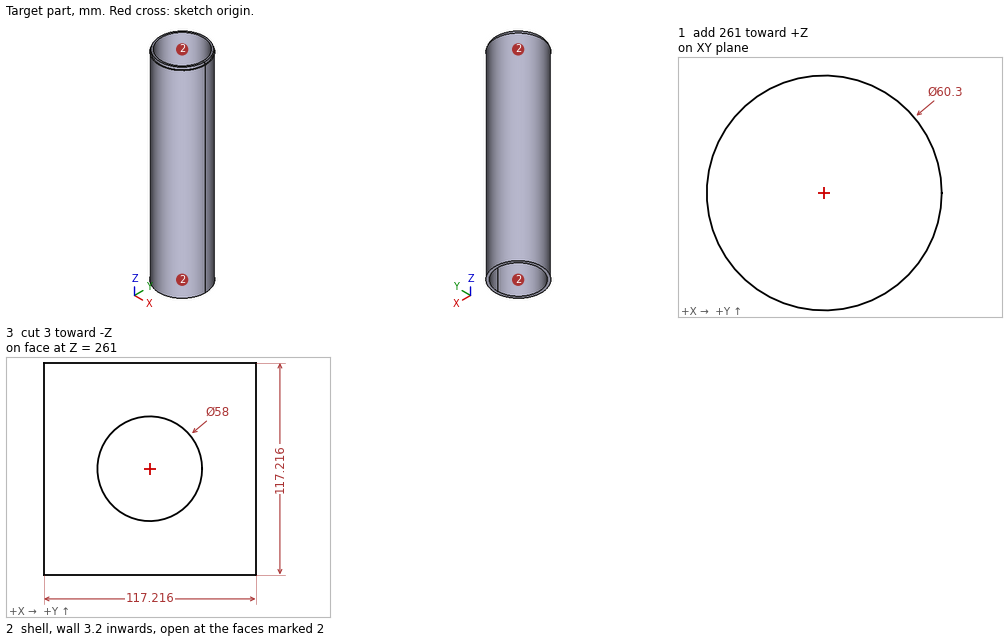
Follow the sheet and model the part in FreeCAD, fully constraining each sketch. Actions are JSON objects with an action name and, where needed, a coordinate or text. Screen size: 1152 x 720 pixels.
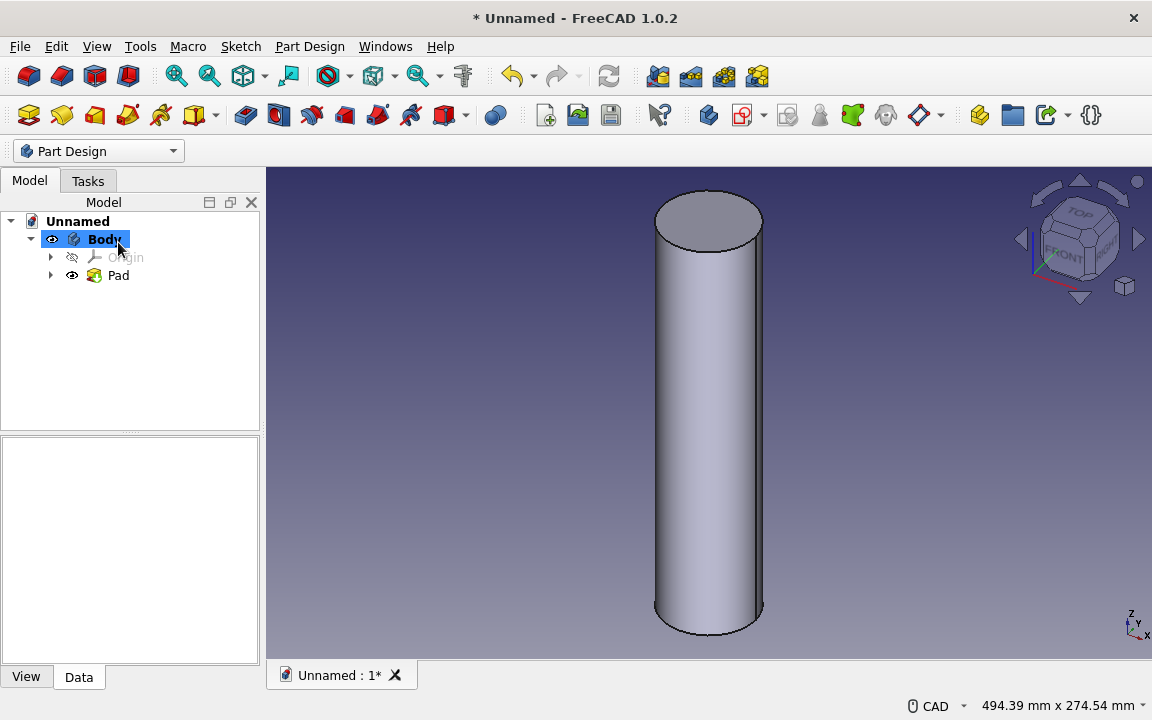
{"action": "left_click", "coordinate": [709, 220]}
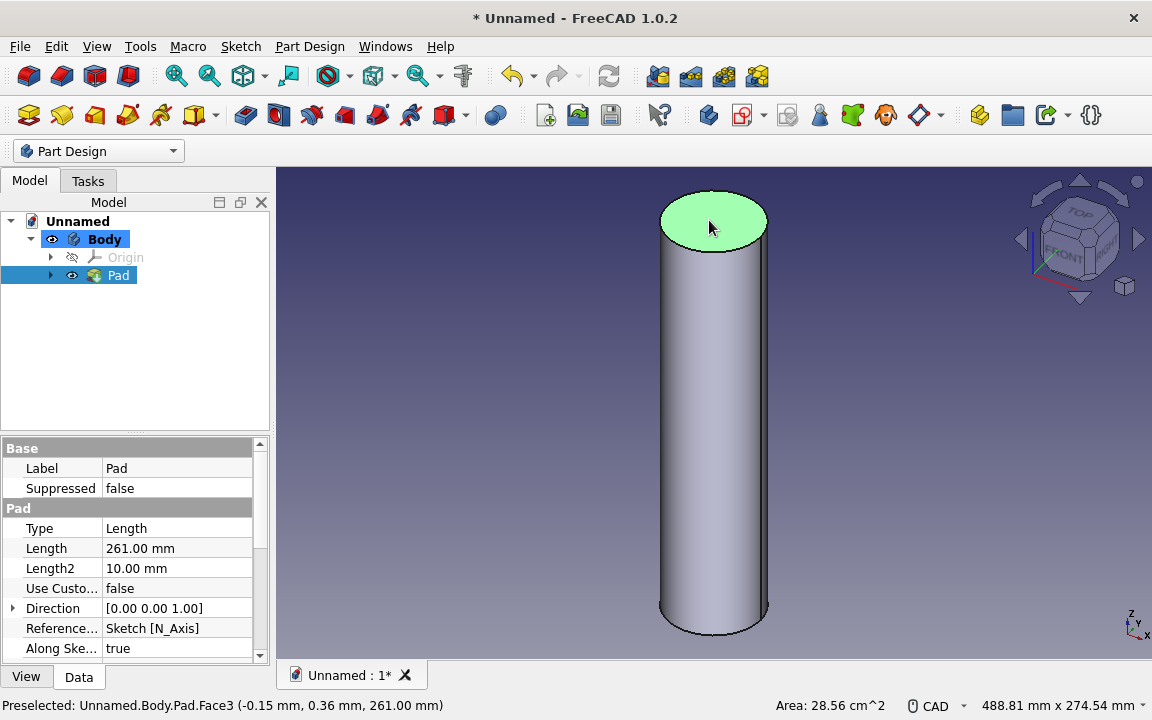
{"action": "key", "text": "0"}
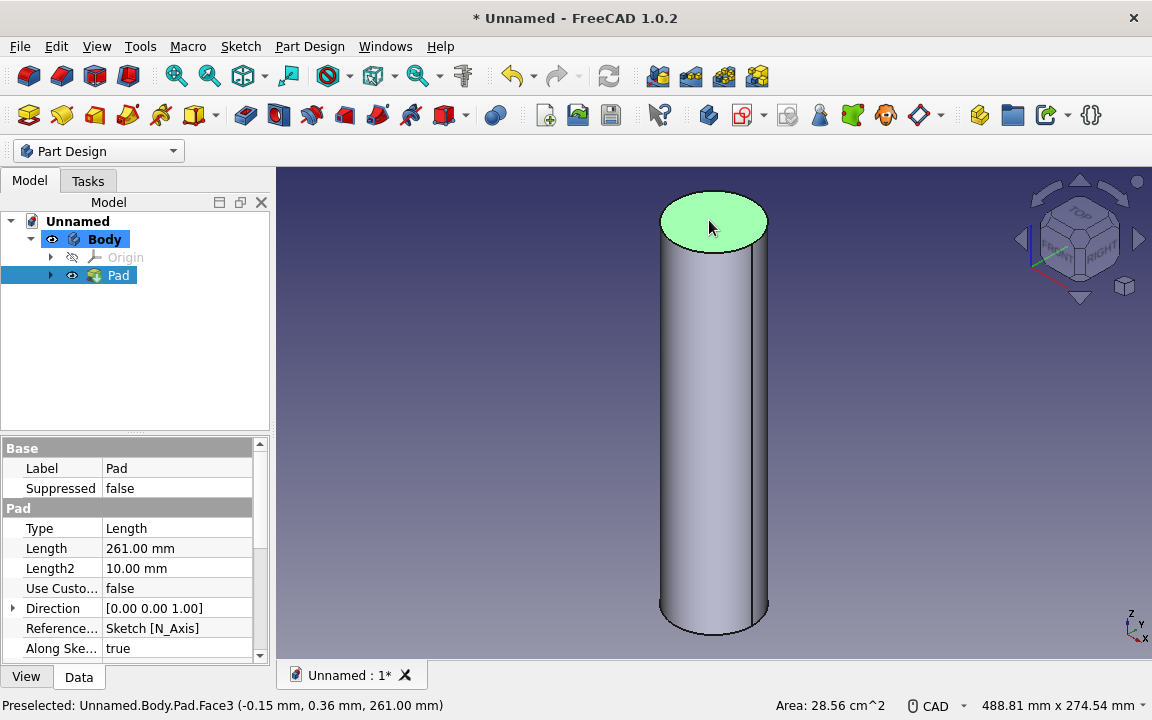
{"action": "key", "text": "2"}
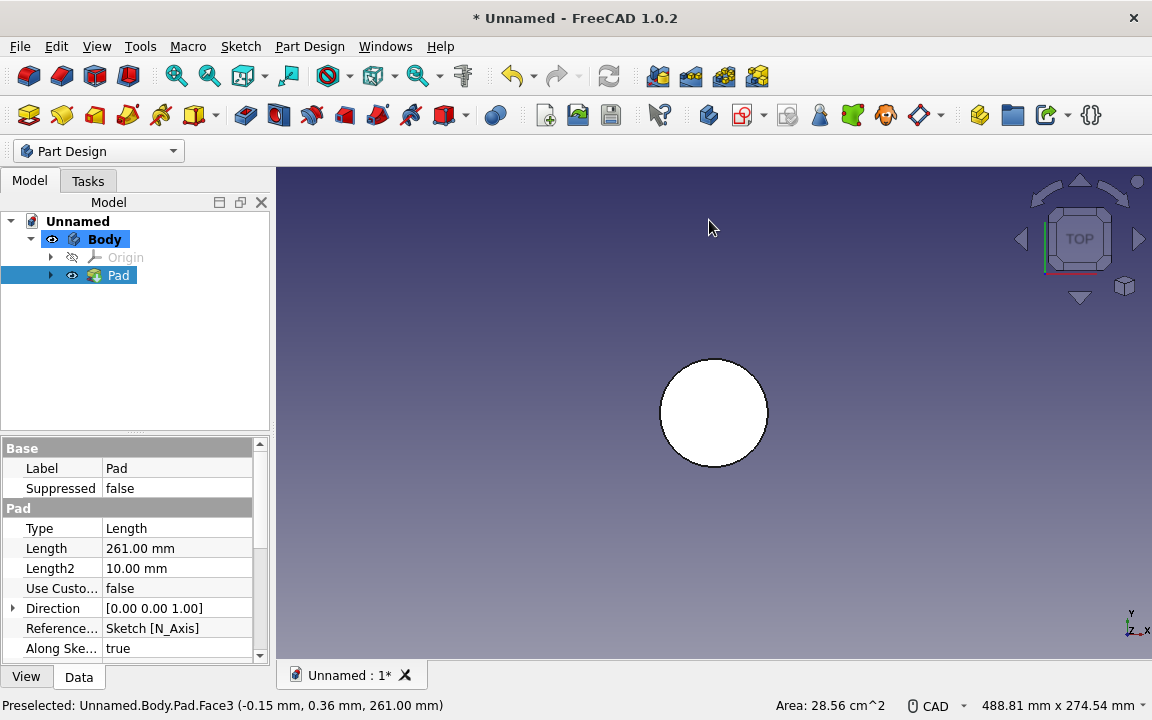
{"action": "left_click", "coordinate": [177, 76]}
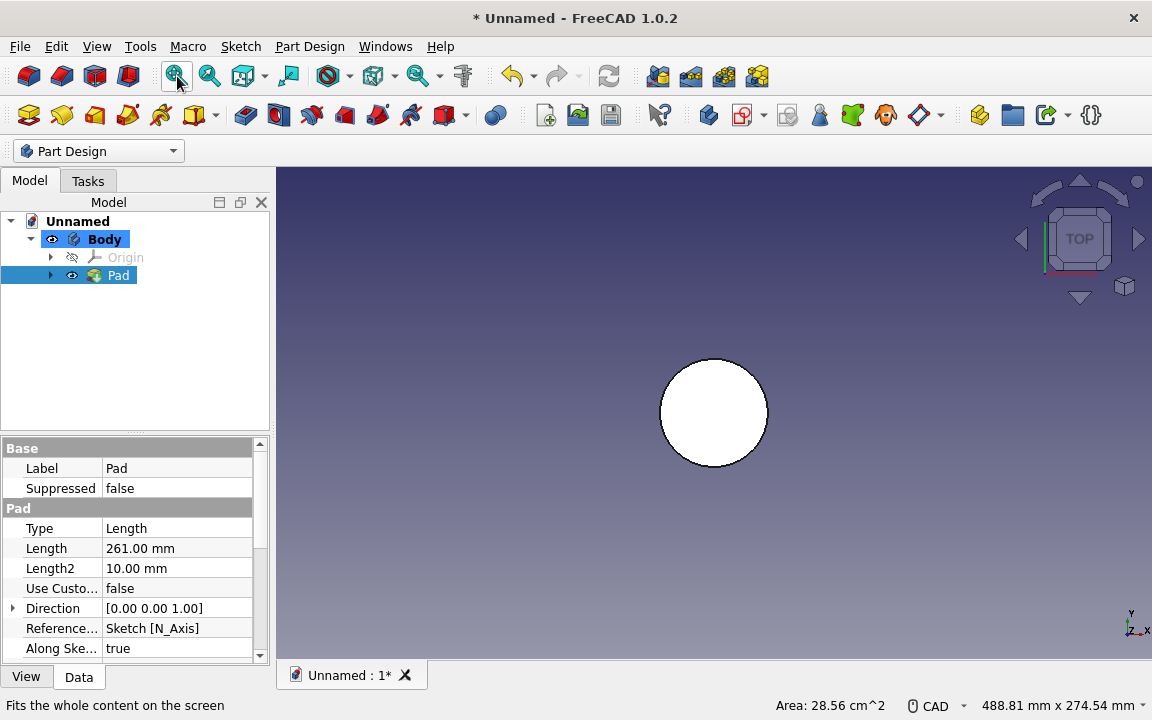
{"action": "key", "text": "1"}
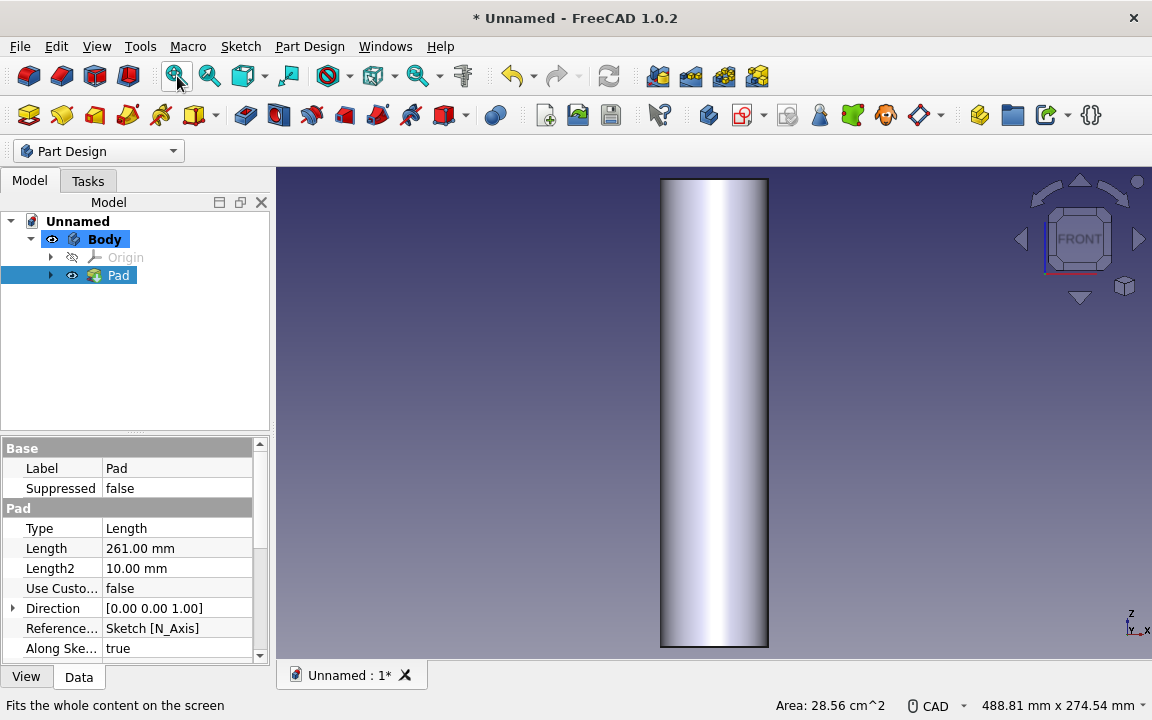
{"action": "key", "text": "3"}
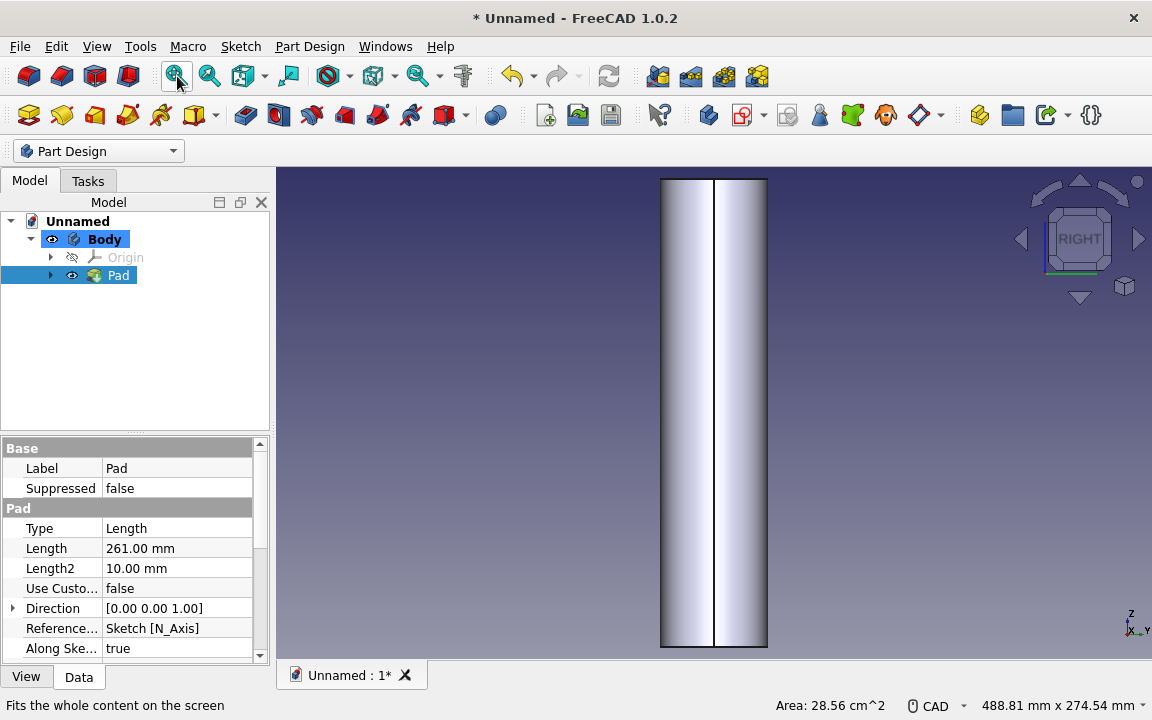
{"action": "key", "text": "5"}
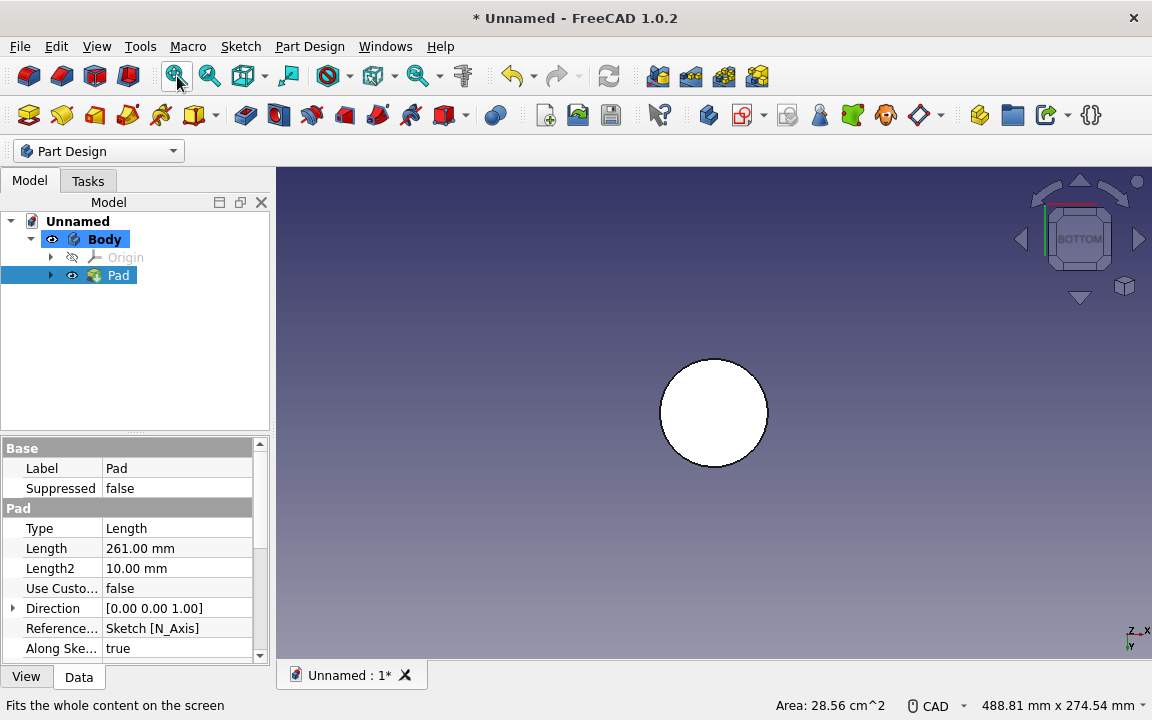
{"action": "key", "text": "v f"}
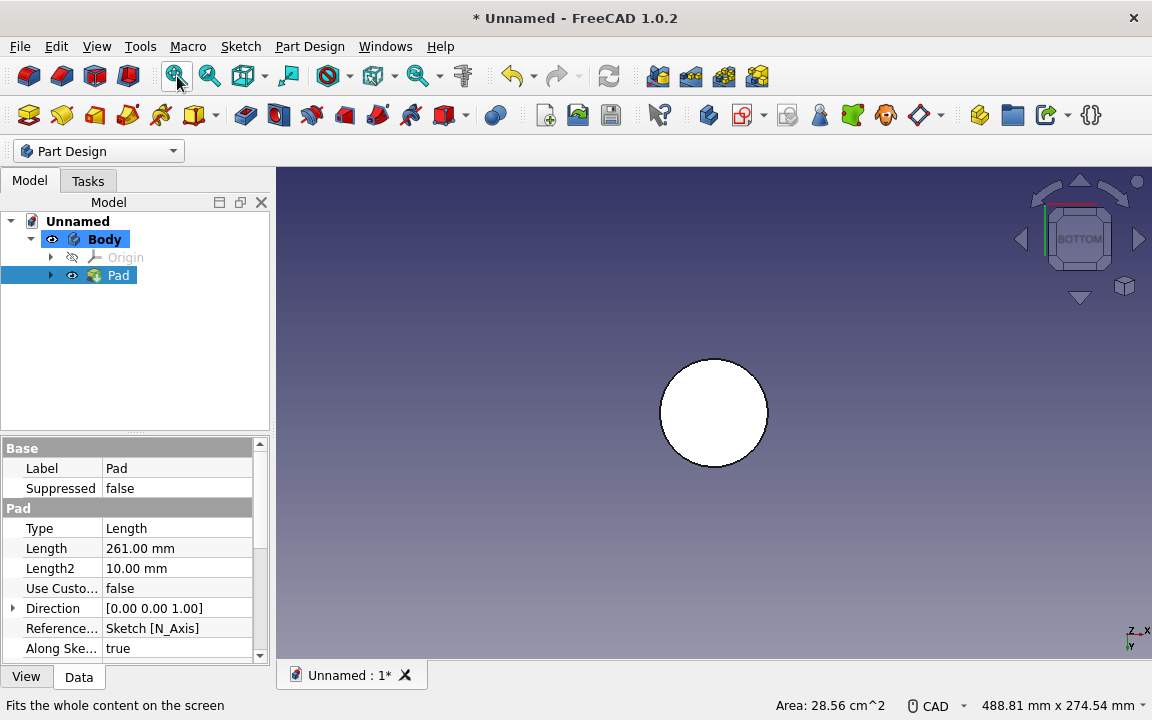
{"action": "left_click", "coordinate": [714, 412], "text": "ctrl"}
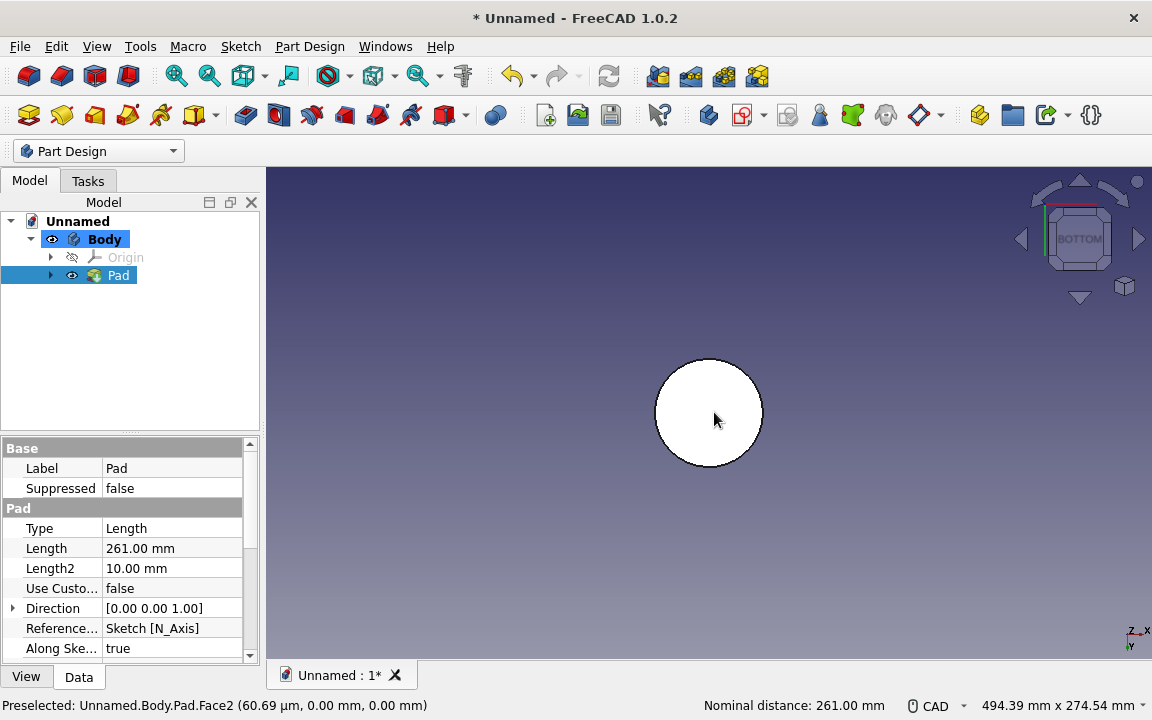
{"action": "left_click", "coordinate": [128, 76]}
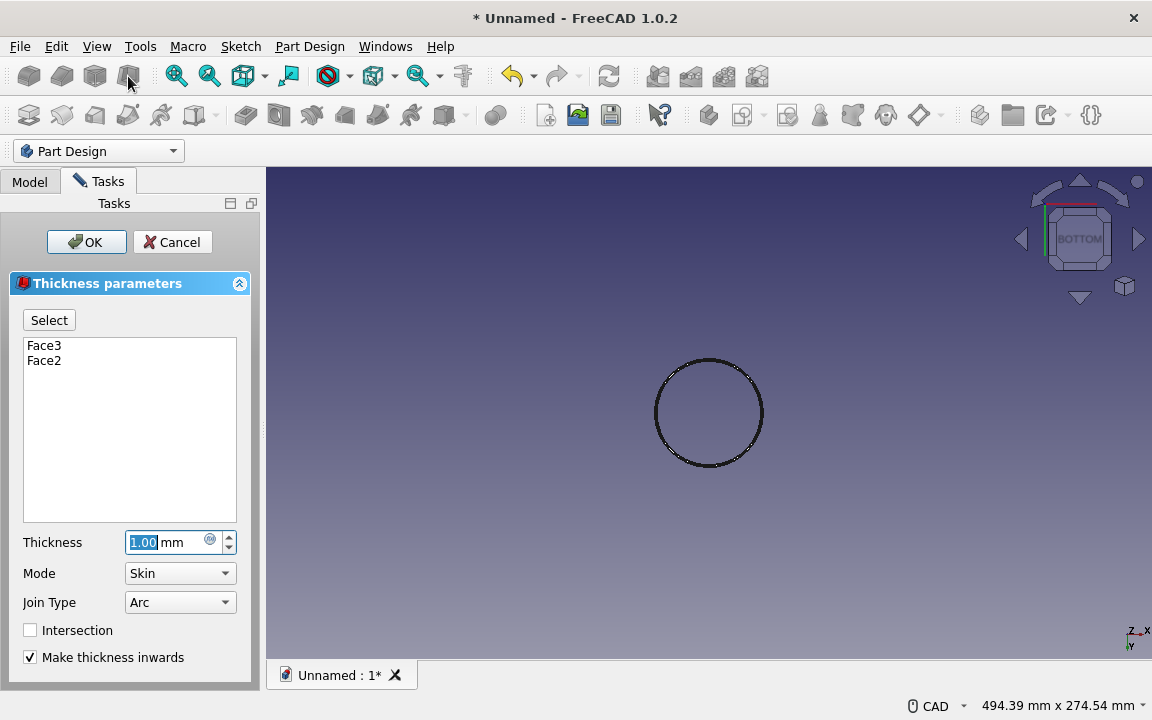
{"action": "type", "text": "3.2"}
{"action": "key", "text": "Tab"}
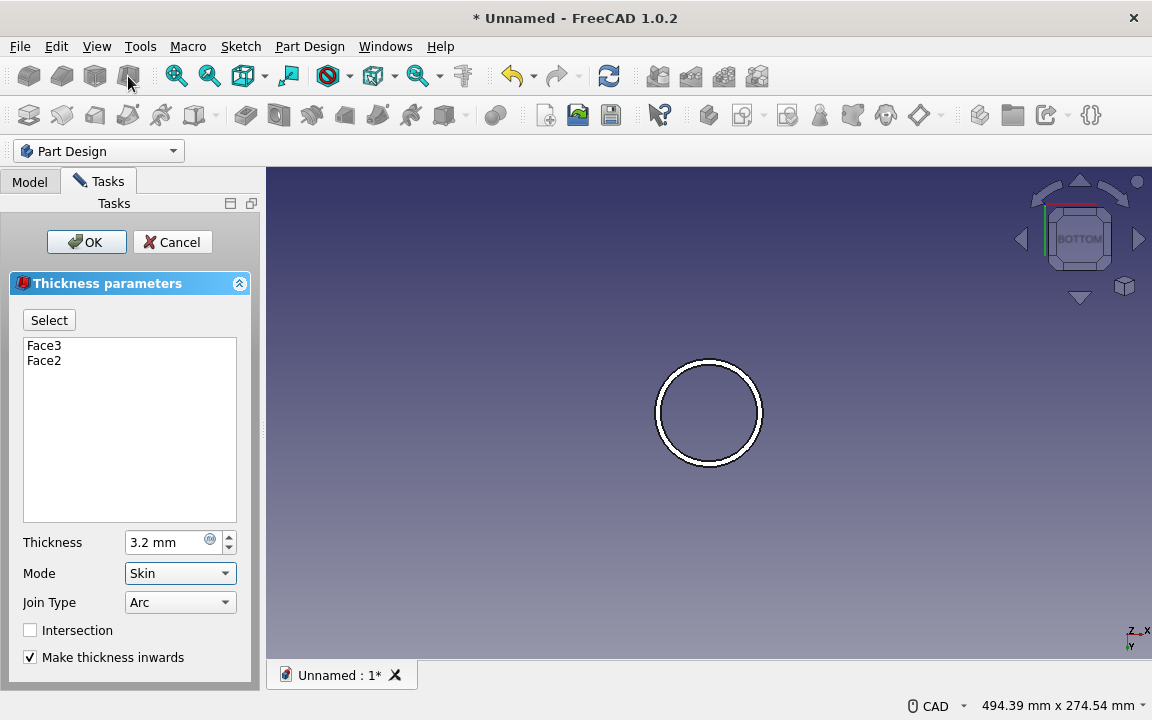
{"action": "left_click", "coordinate": [181, 602]}